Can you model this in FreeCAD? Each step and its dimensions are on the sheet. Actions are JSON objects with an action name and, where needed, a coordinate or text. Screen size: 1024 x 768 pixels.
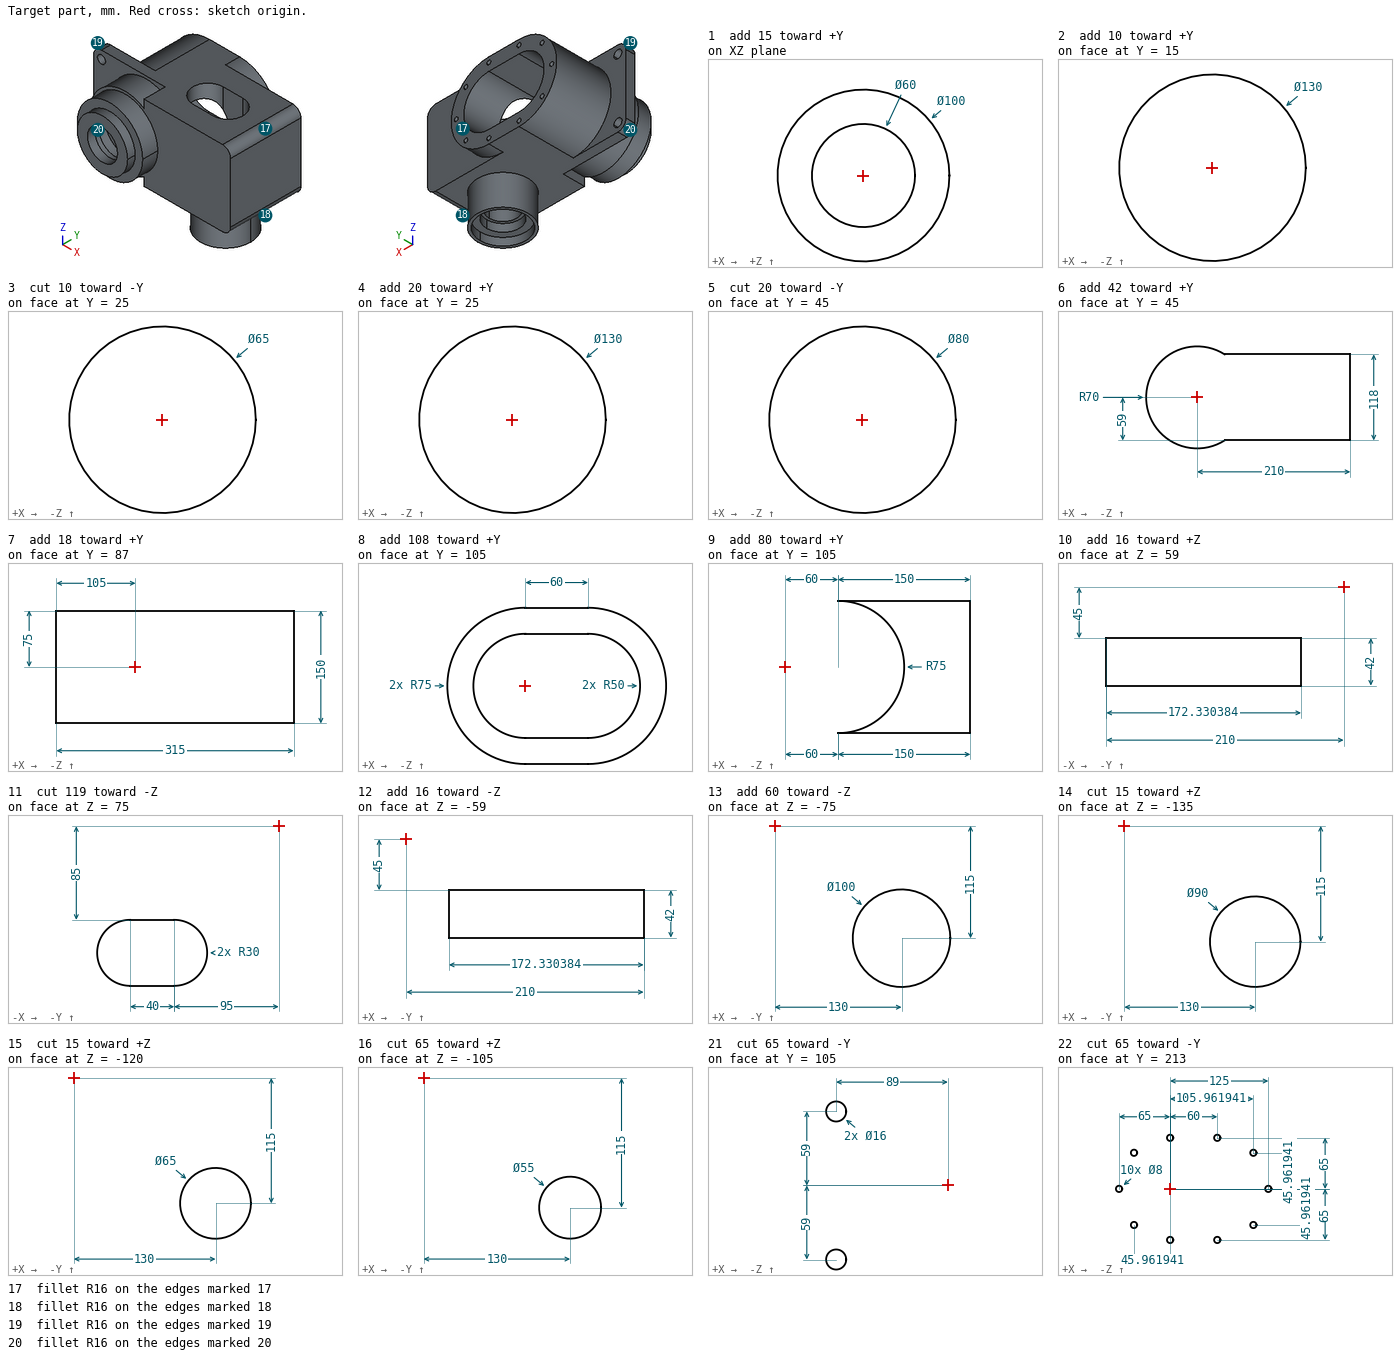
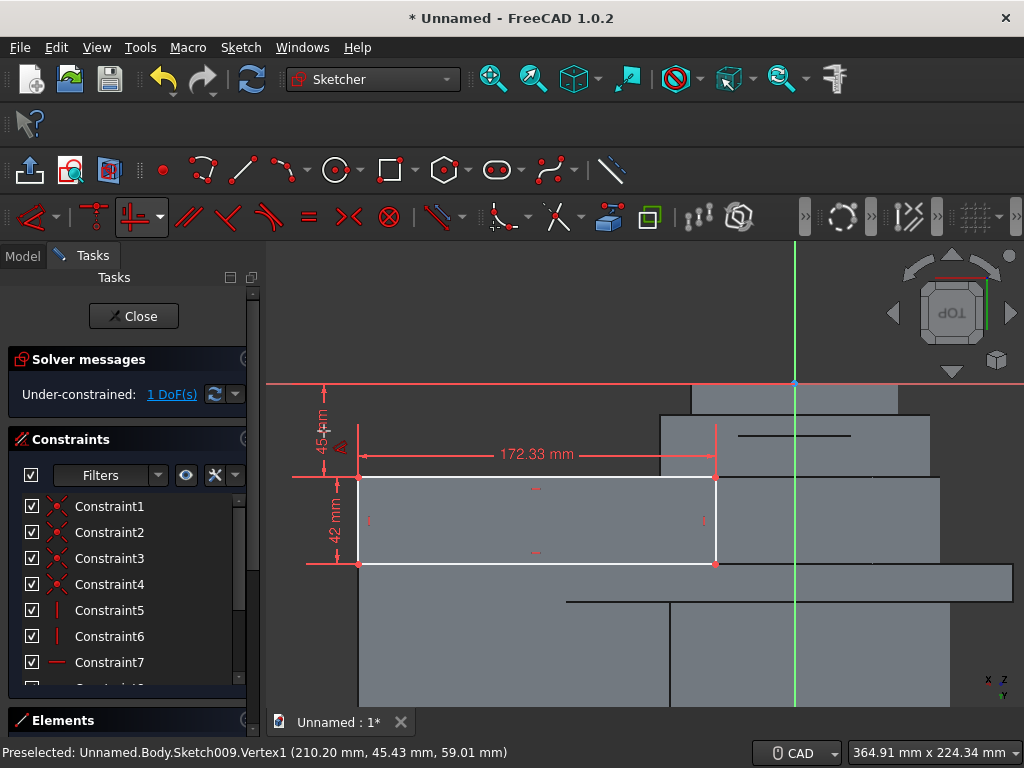
{"action": "left_click", "coordinate": [358, 477]}
{"action": "left_click", "coordinate": [576, 350]}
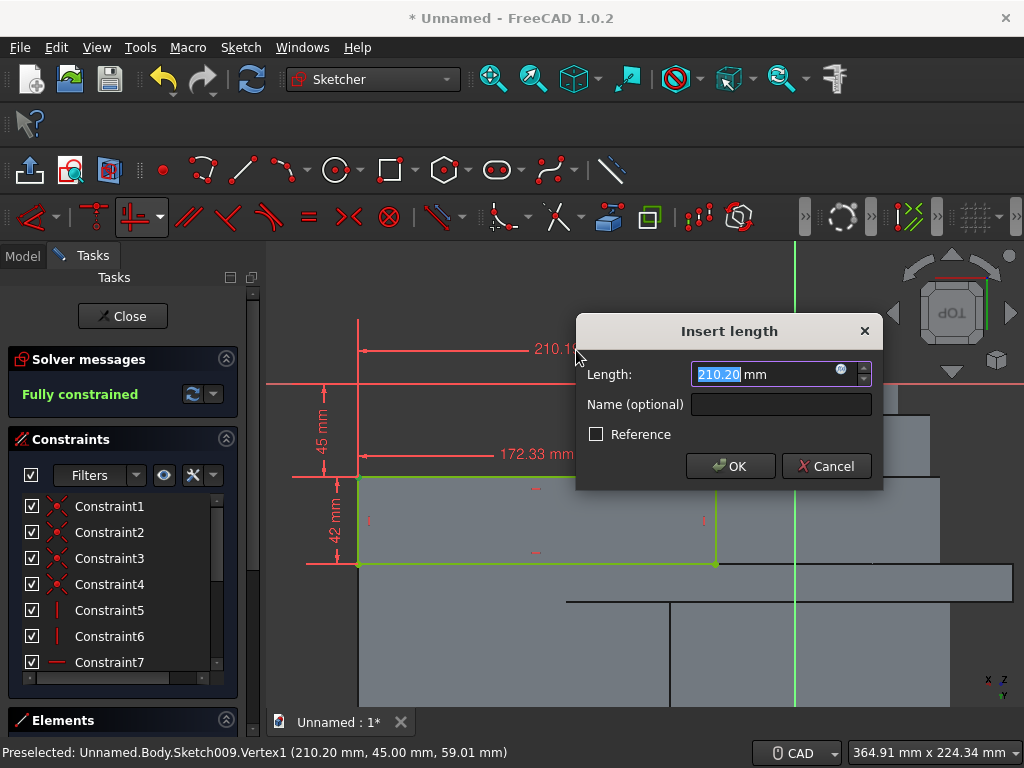
{"action": "type", "text": "210"}
{"action": "key", "text": "Return"}
{"action": "key", "text": "Escape"}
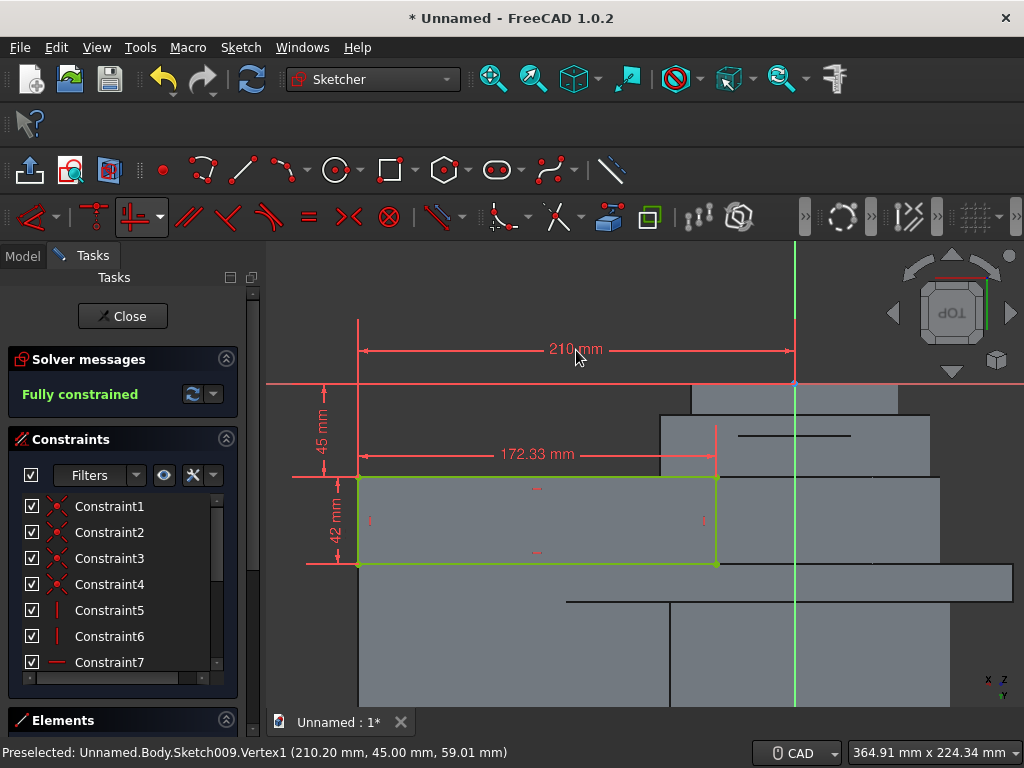
{"action": "left_click", "coordinate": [123, 316]}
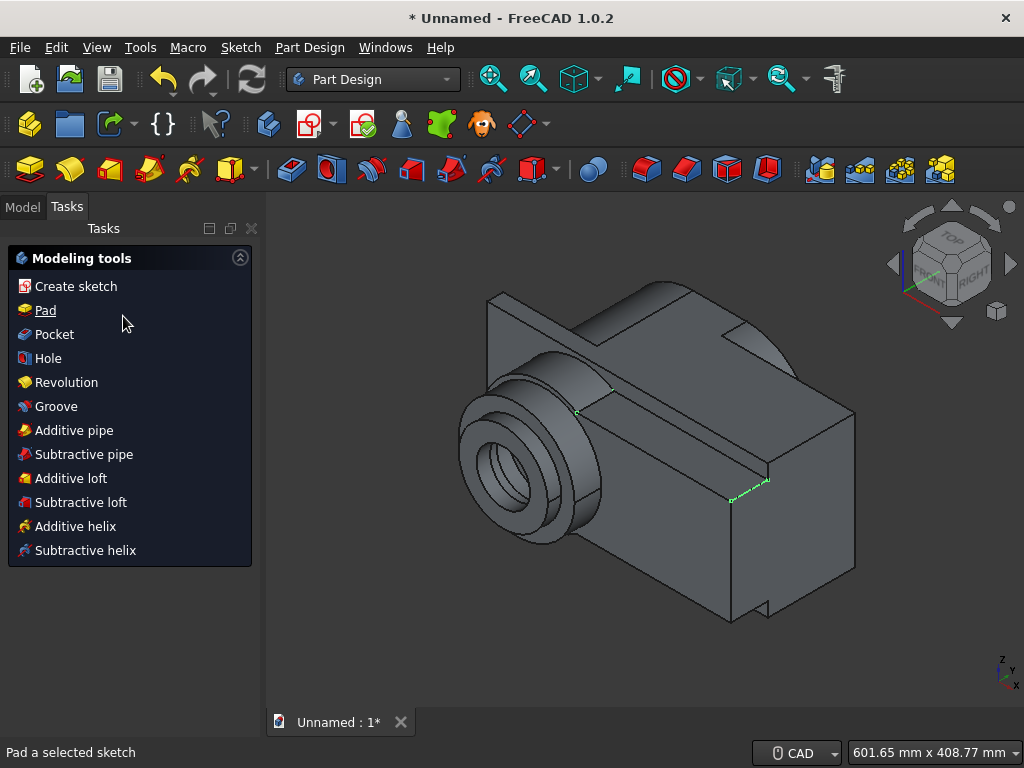
{"action": "left_click", "coordinate": [30, 170]}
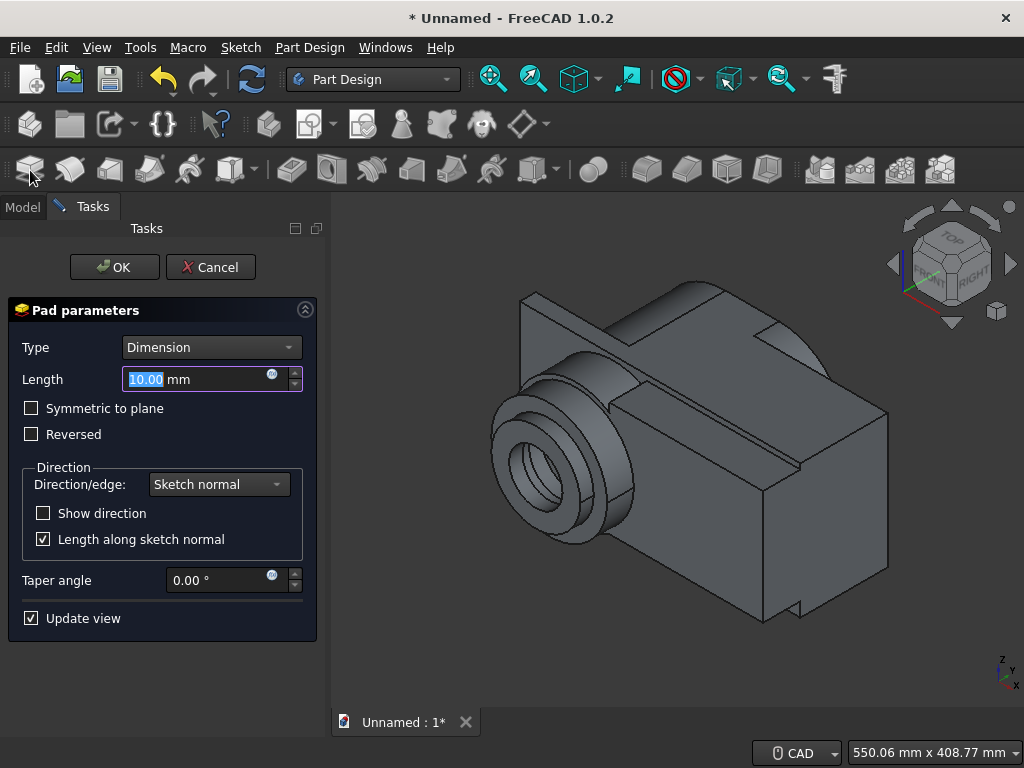
{"action": "type", "text": "16"}
{"action": "key", "text": "Tab"}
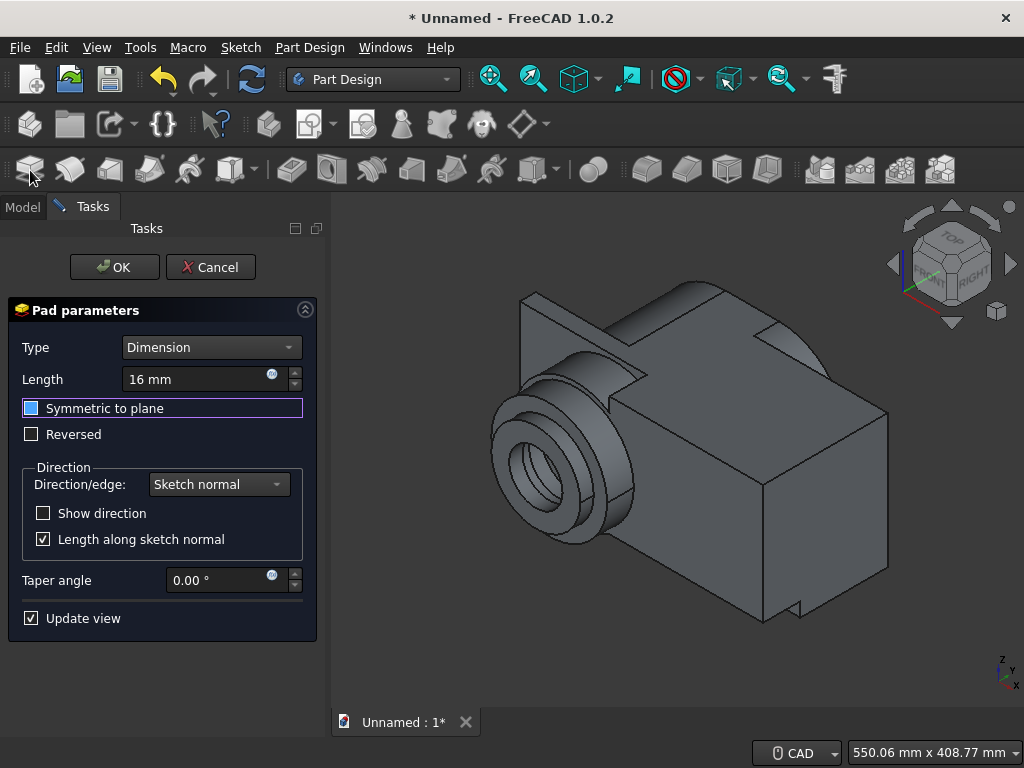
{"action": "left_click", "coordinate": [115, 267]}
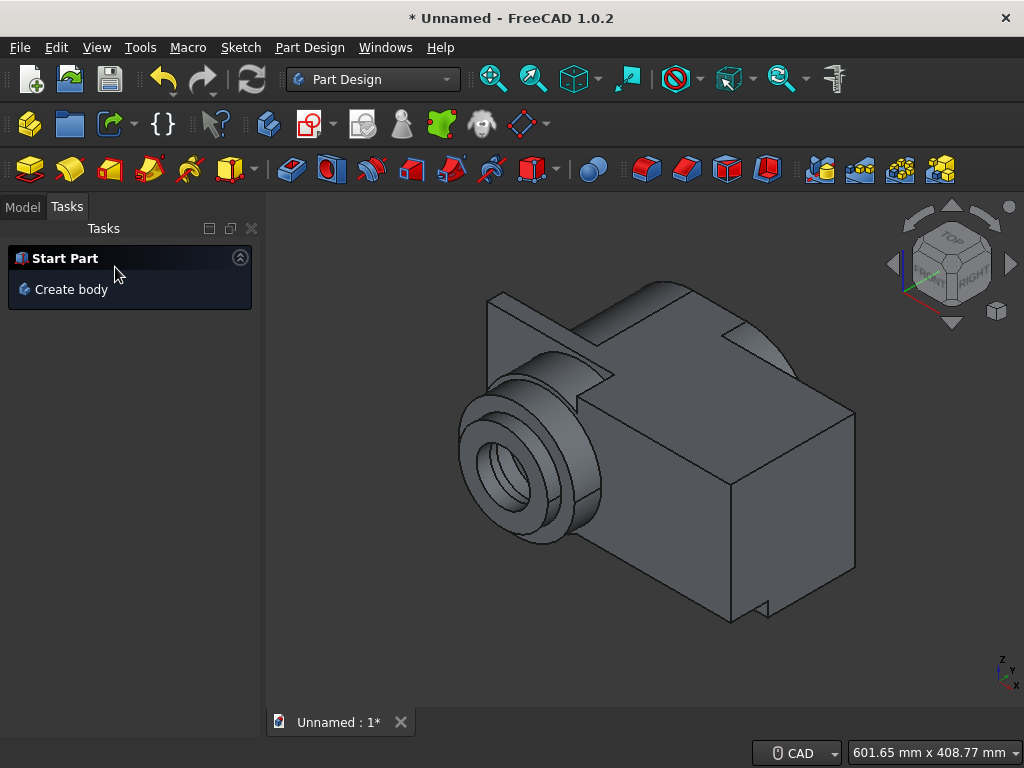
{"action": "left_click", "coordinate": [724, 418]}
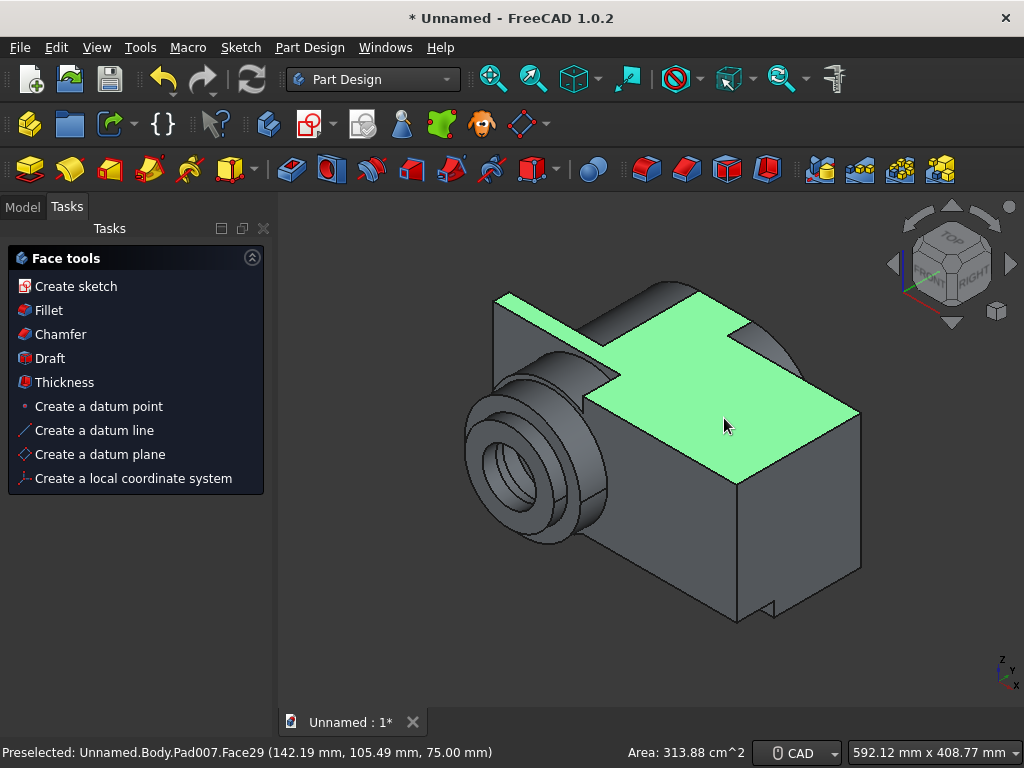
{"action": "left_click", "coordinate": [310, 124]}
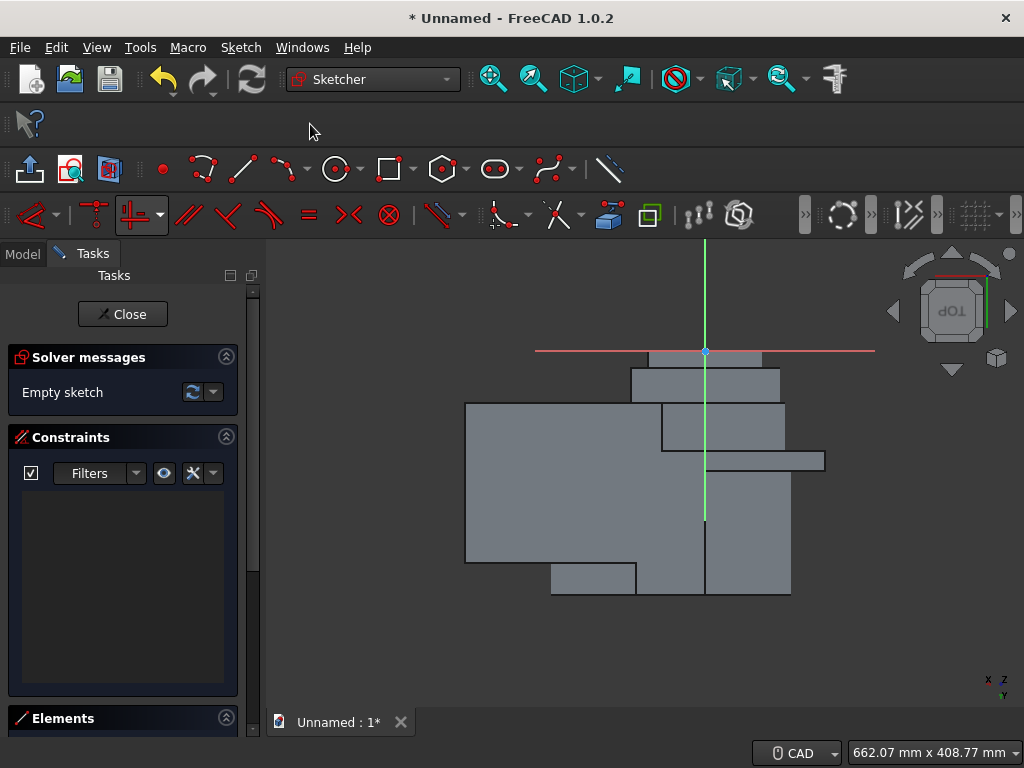
{"action": "scroll", "coordinate": [652, 387], "scroll_direction": "up", "scroll_amount": 3}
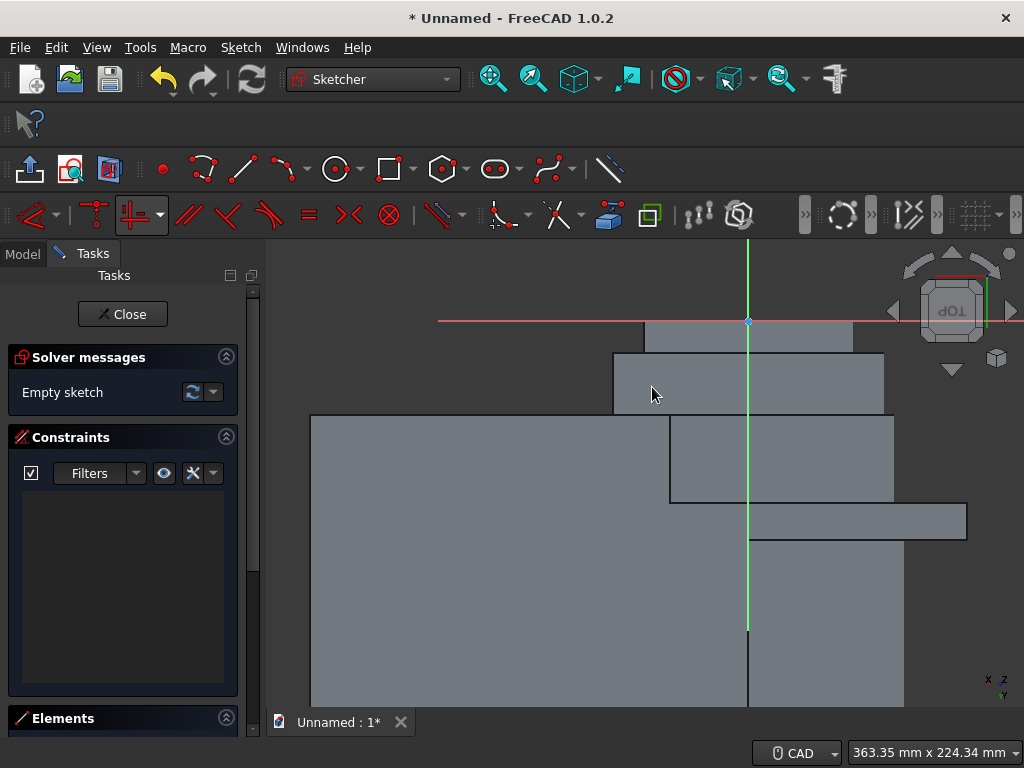
{"action": "left_click", "coordinate": [496, 170]}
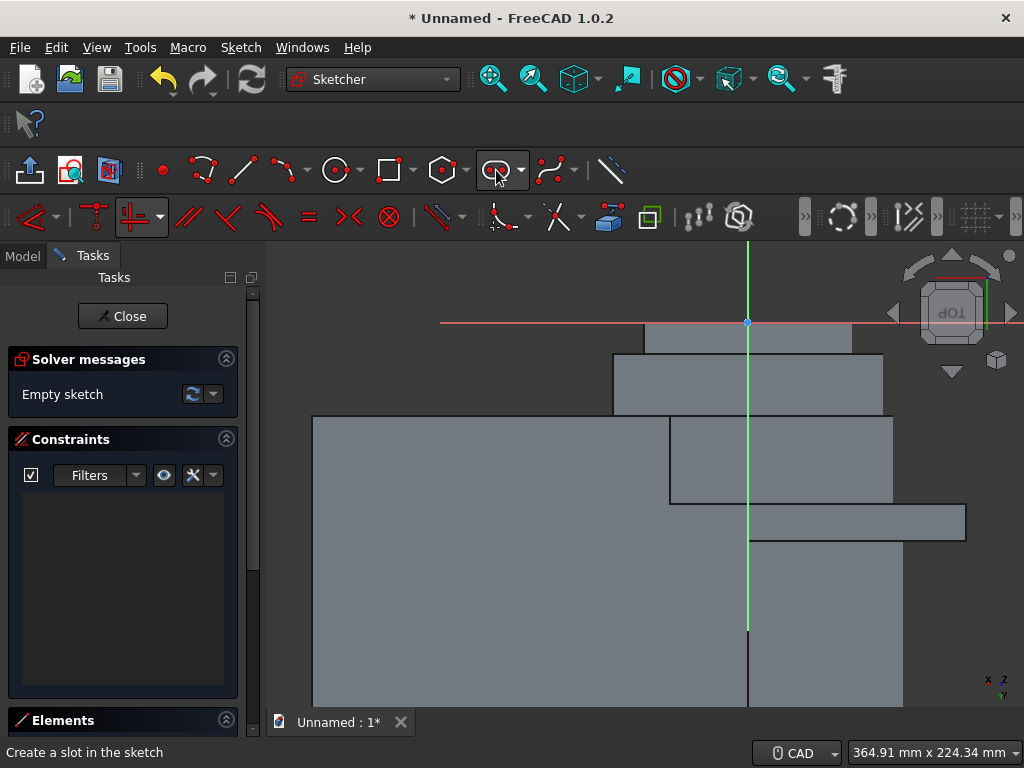
{"action": "left_click", "coordinate": [467, 562]}